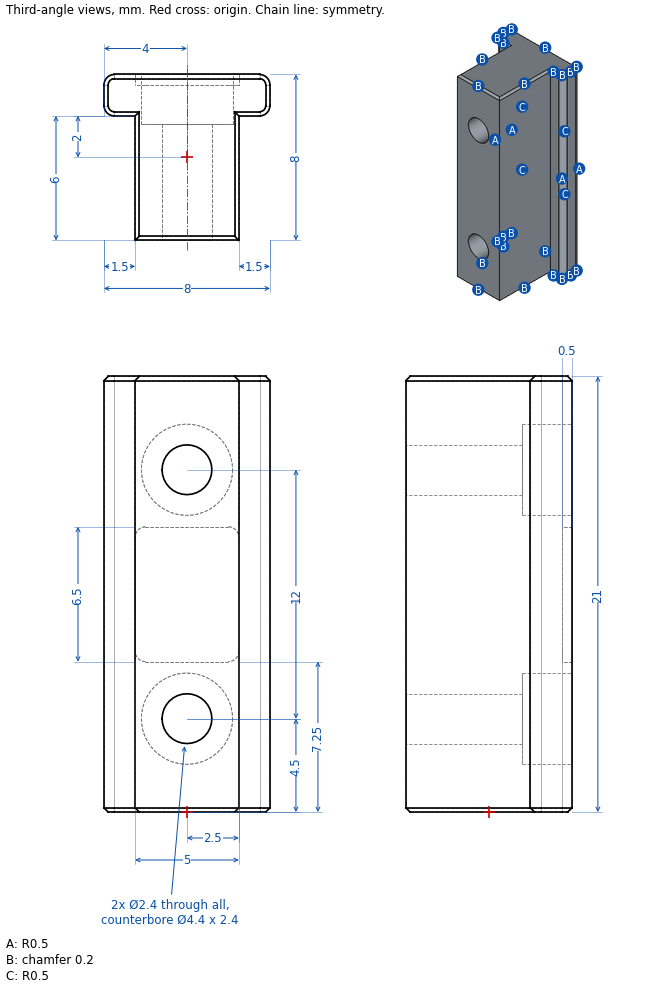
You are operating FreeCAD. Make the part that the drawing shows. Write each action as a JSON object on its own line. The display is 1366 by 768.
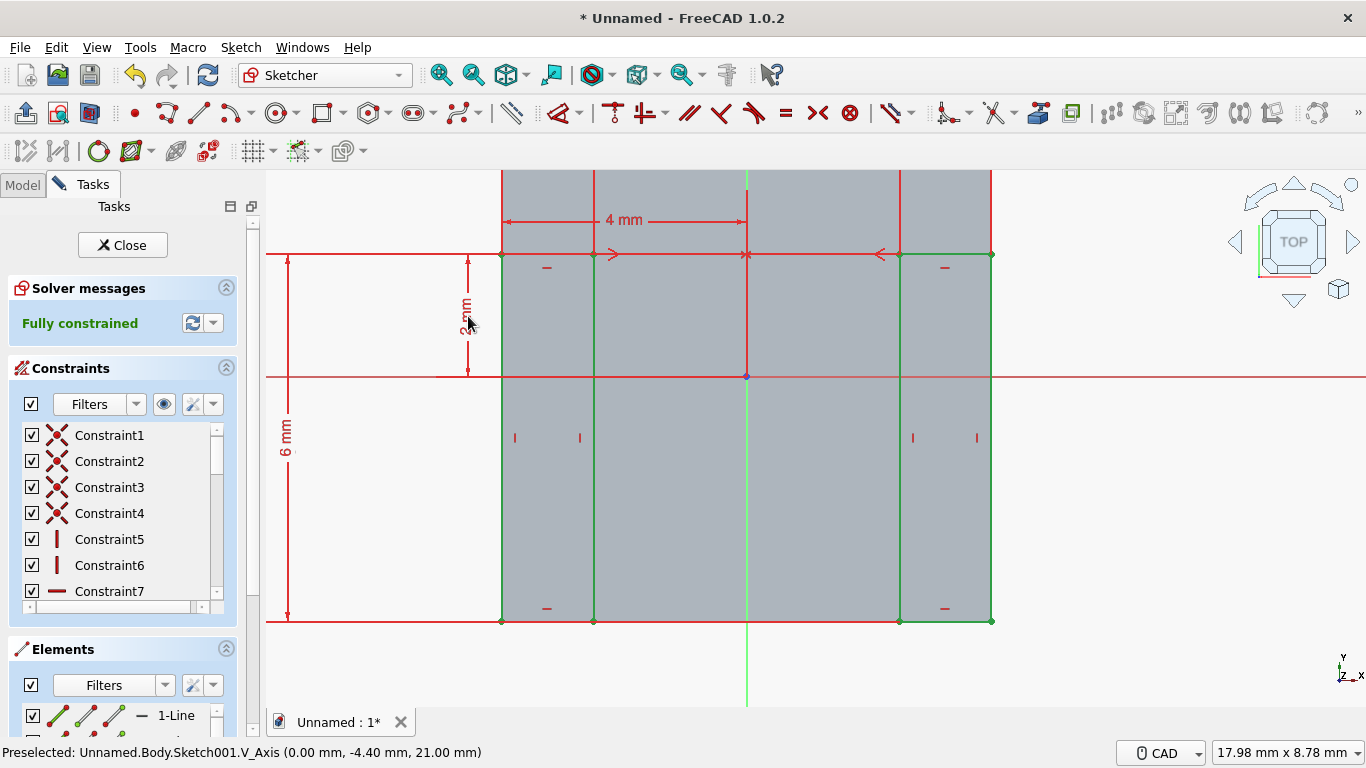
{"action": "left_click", "coordinate": [123, 245]}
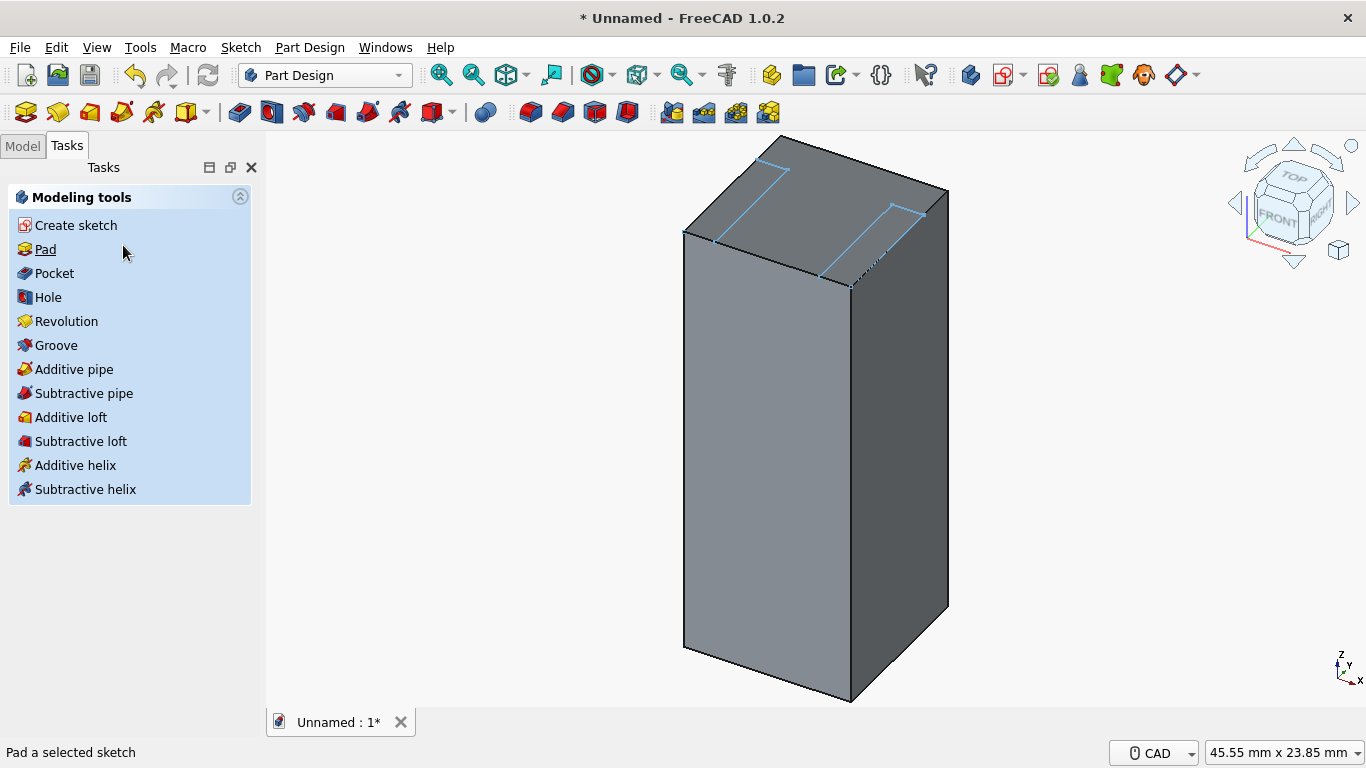
{"action": "left_click", "coordinate": [240, 112]}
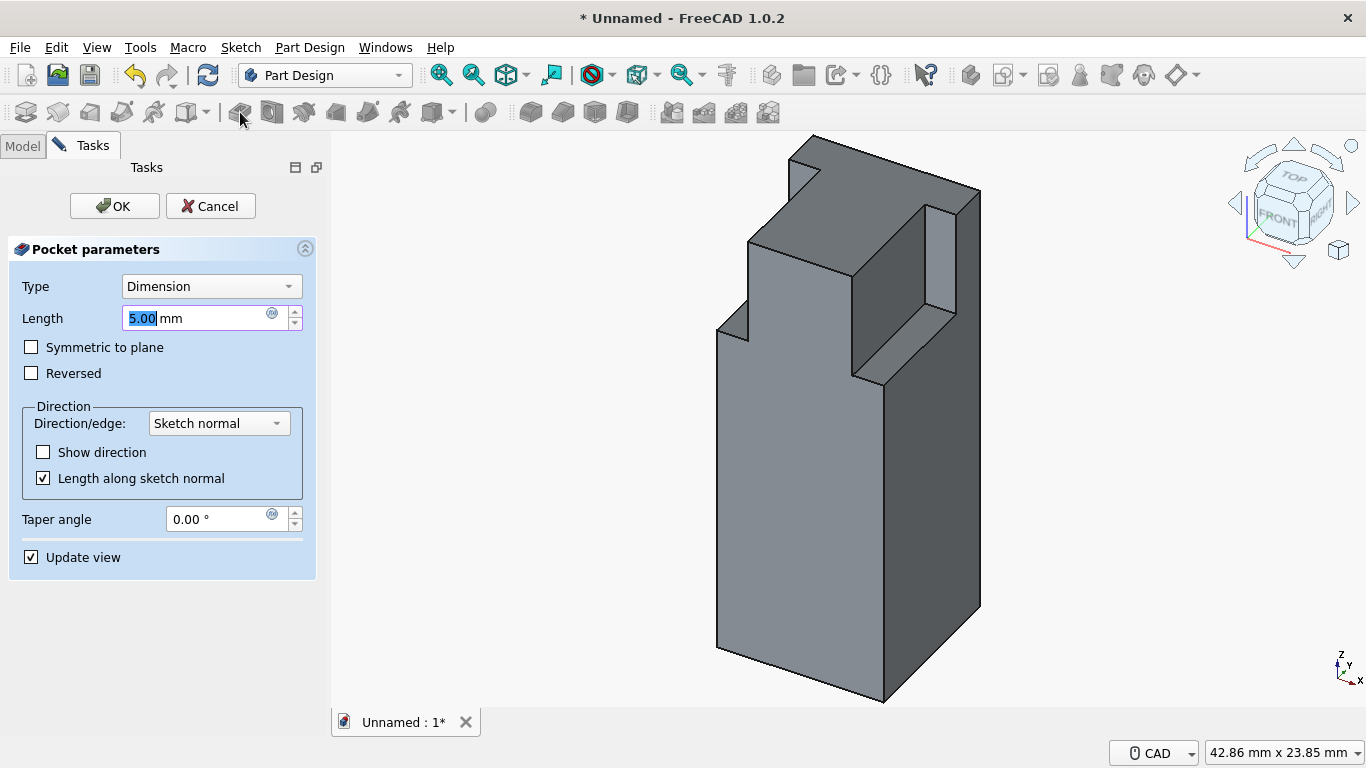
{"action": "left_click", "coordinate": [212, 286]}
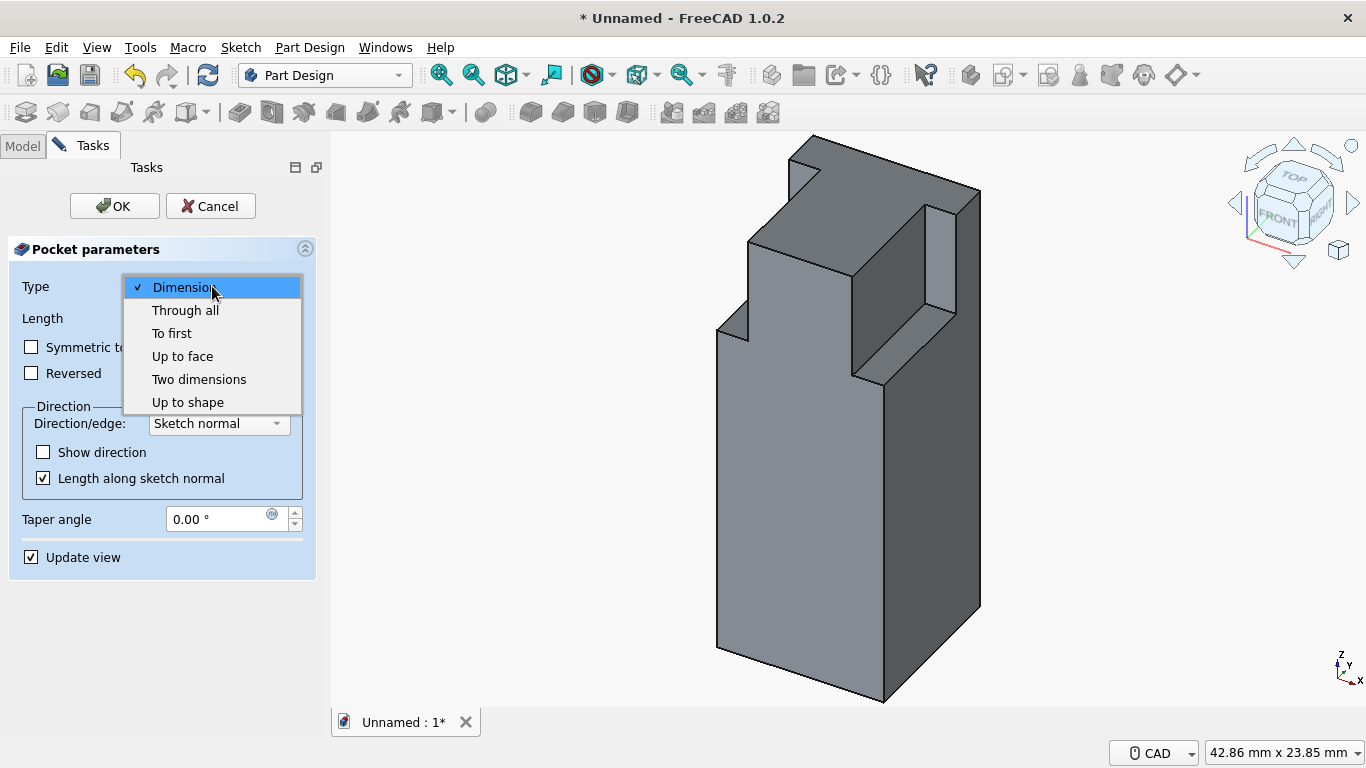
{"action": "left_click", "coordinate": [212, 310]}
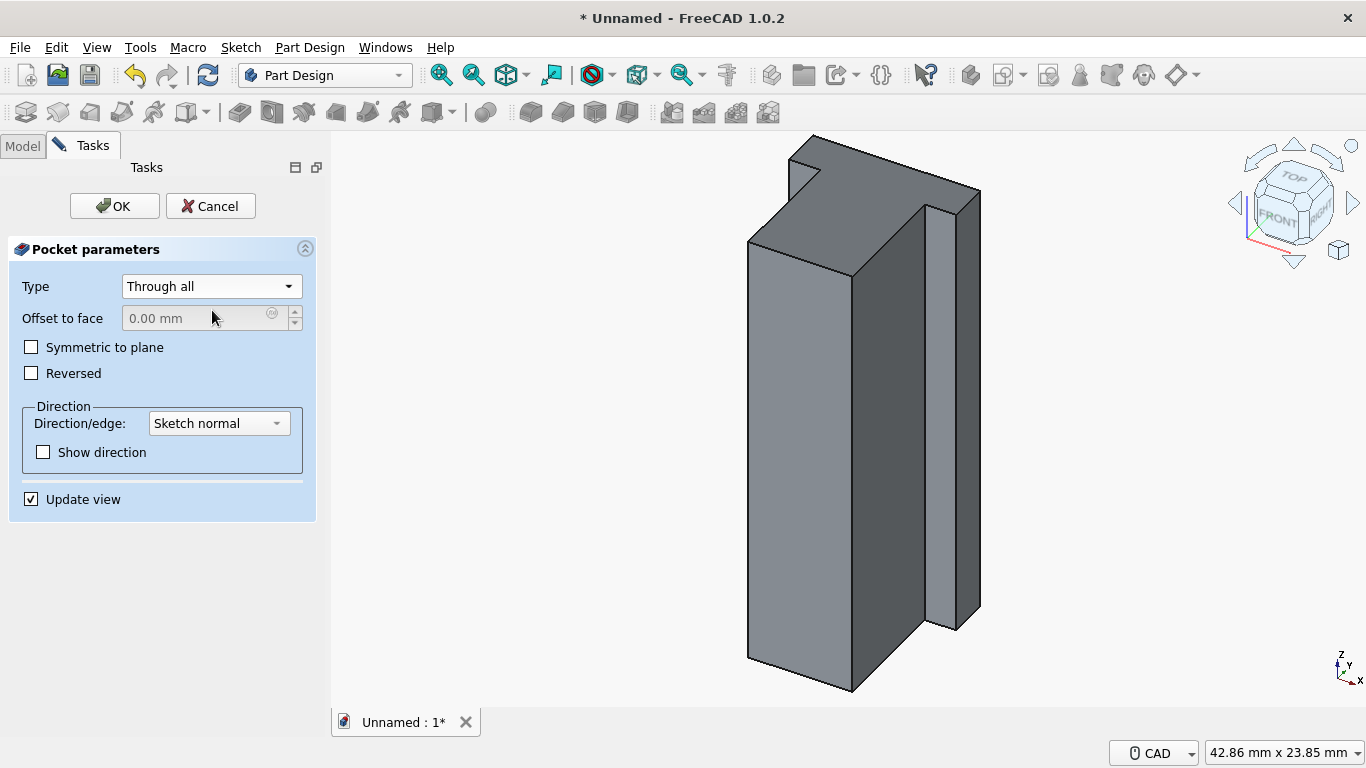
{"action": "left_click", "coordinate": [115, 206]}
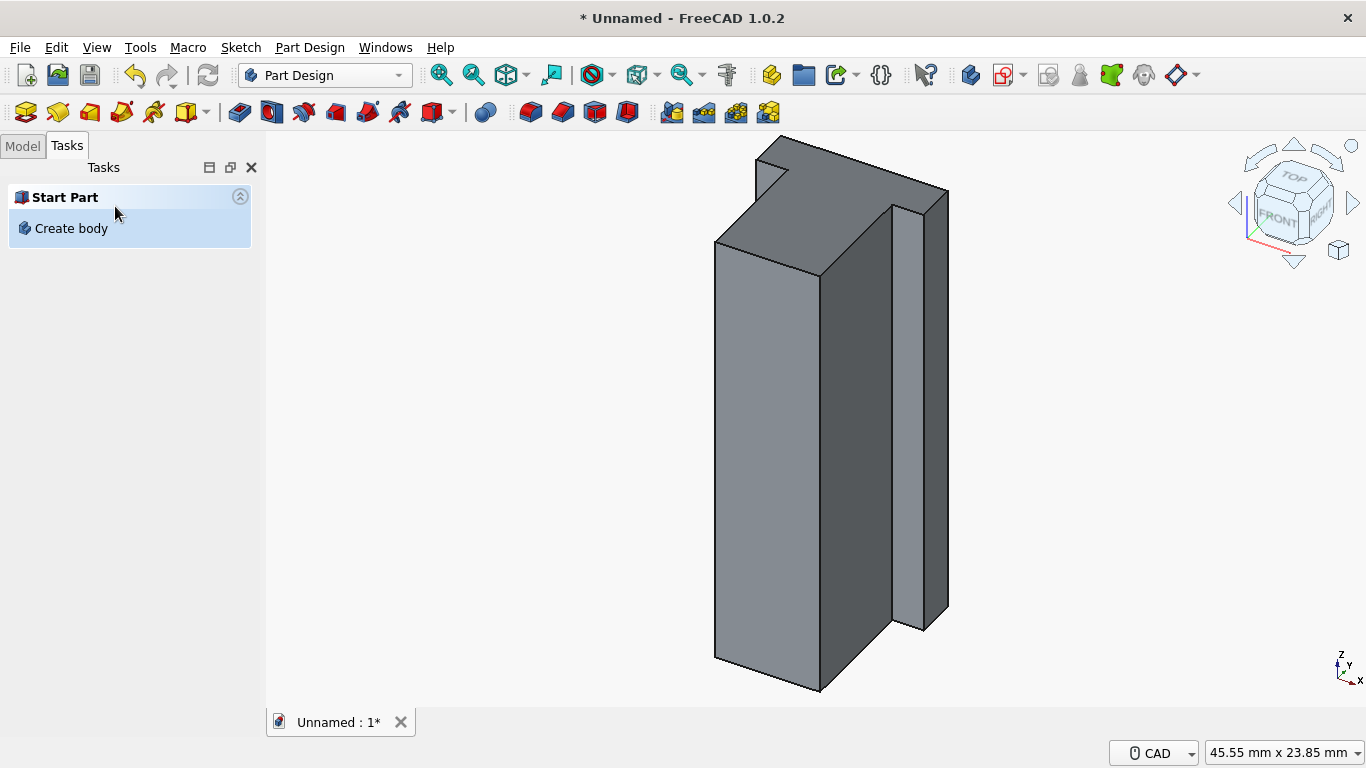
{"action": "left_click", "coordinate": [924, 422]}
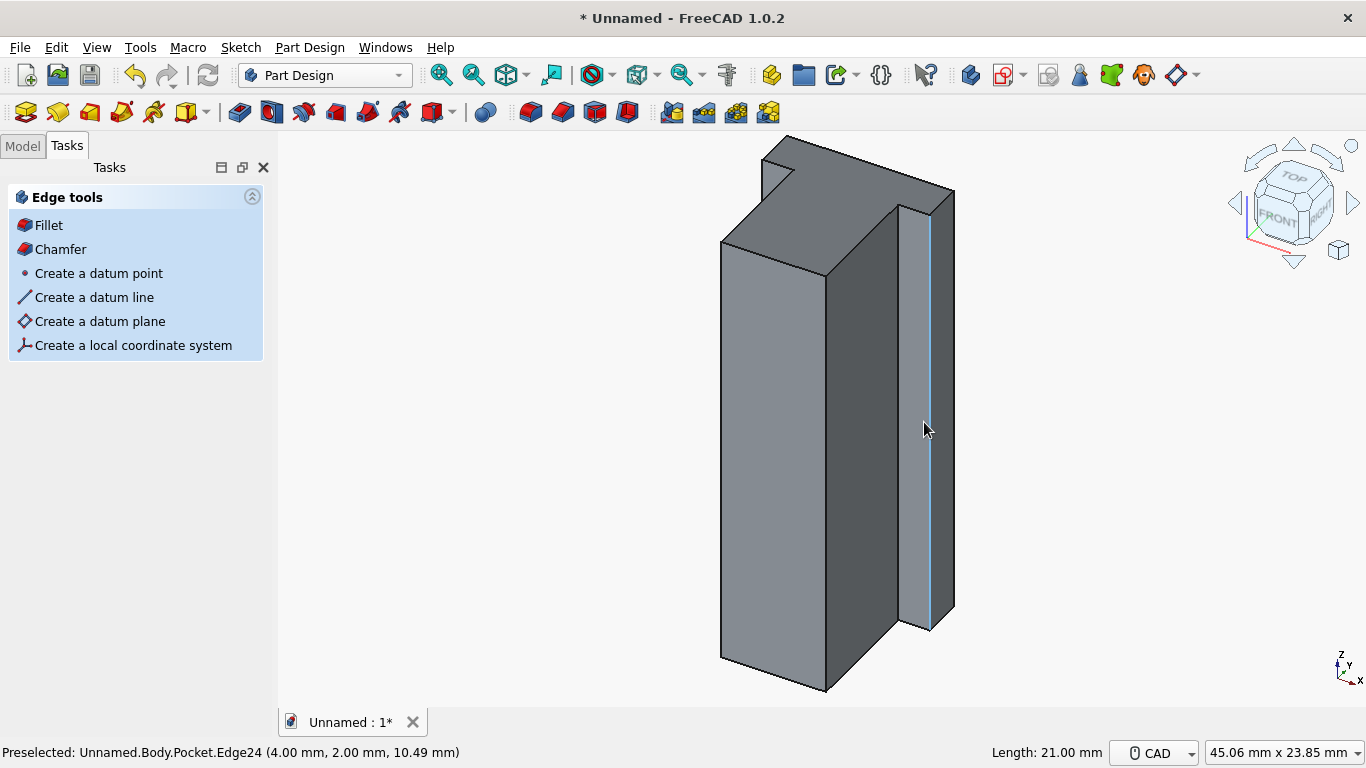
{"action": "key", "text": "0"}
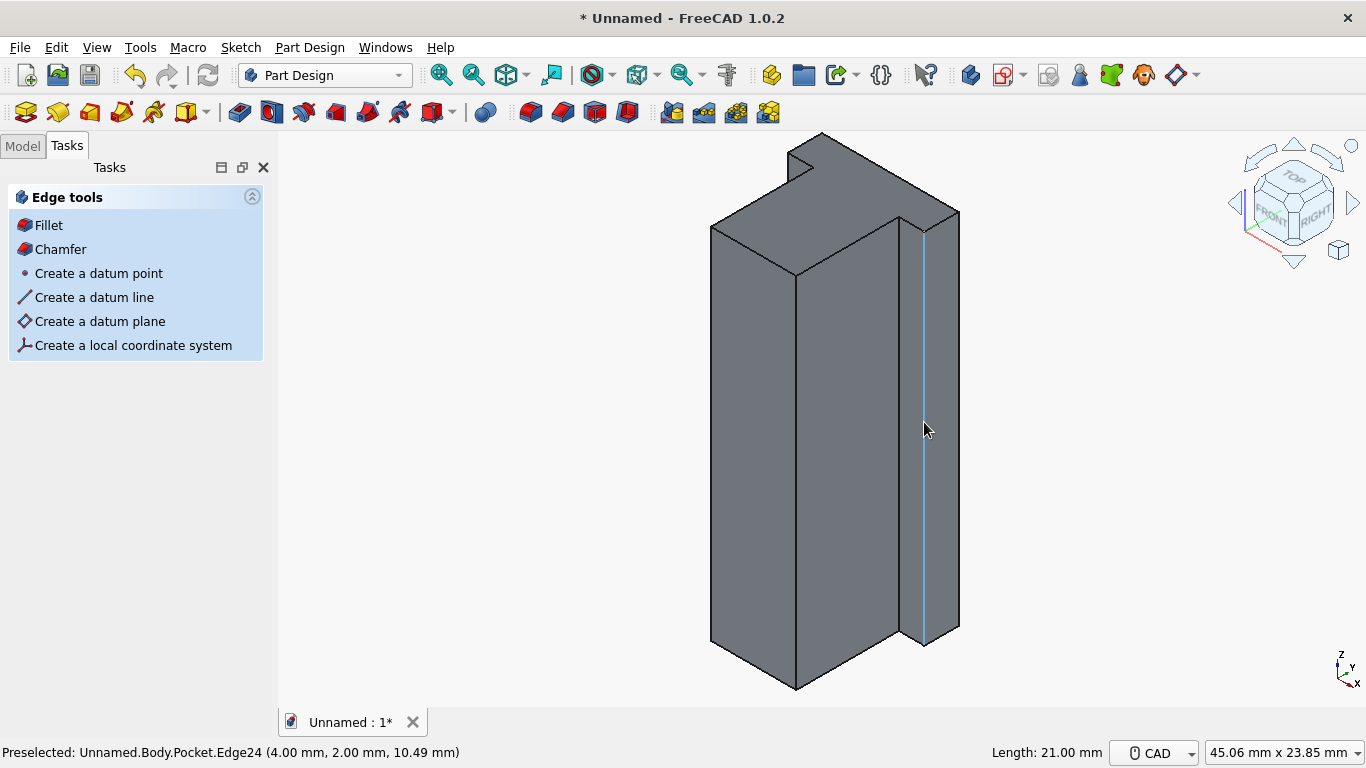
{"action": "key", "text": "2"}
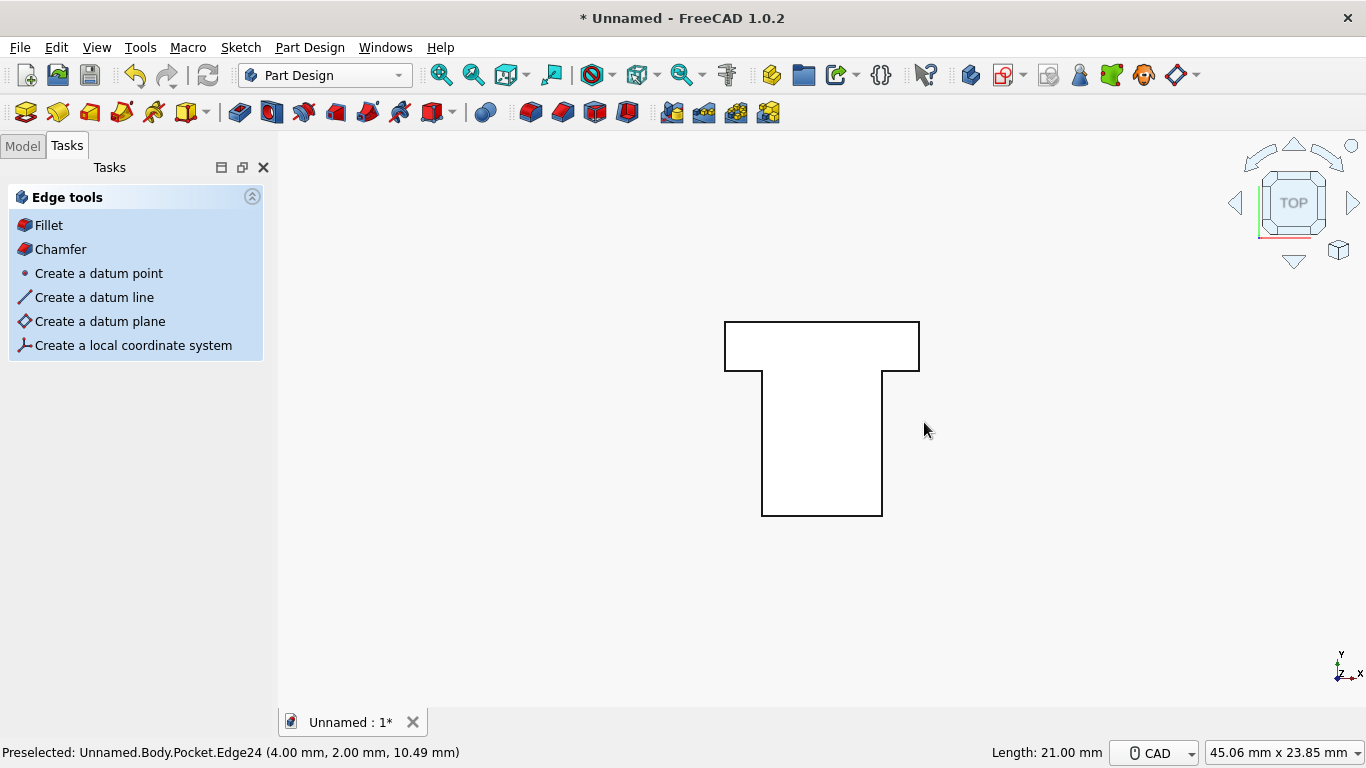
{"action": "left_click", "coordinate": [442, 76]}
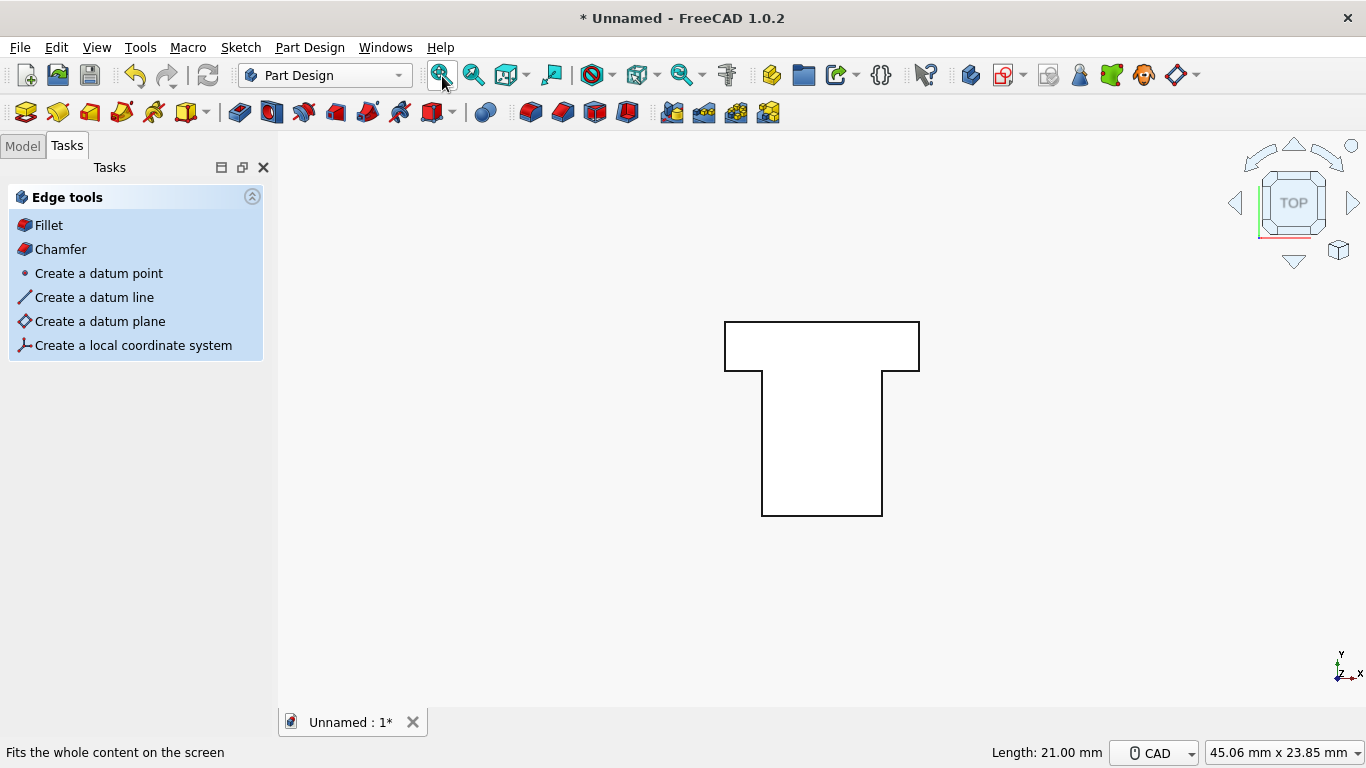
{"action": "key", "text": "1"}